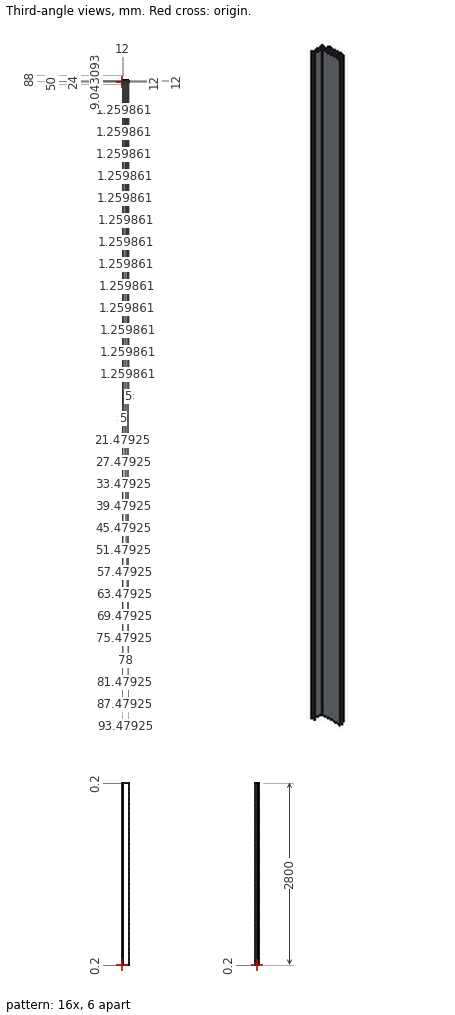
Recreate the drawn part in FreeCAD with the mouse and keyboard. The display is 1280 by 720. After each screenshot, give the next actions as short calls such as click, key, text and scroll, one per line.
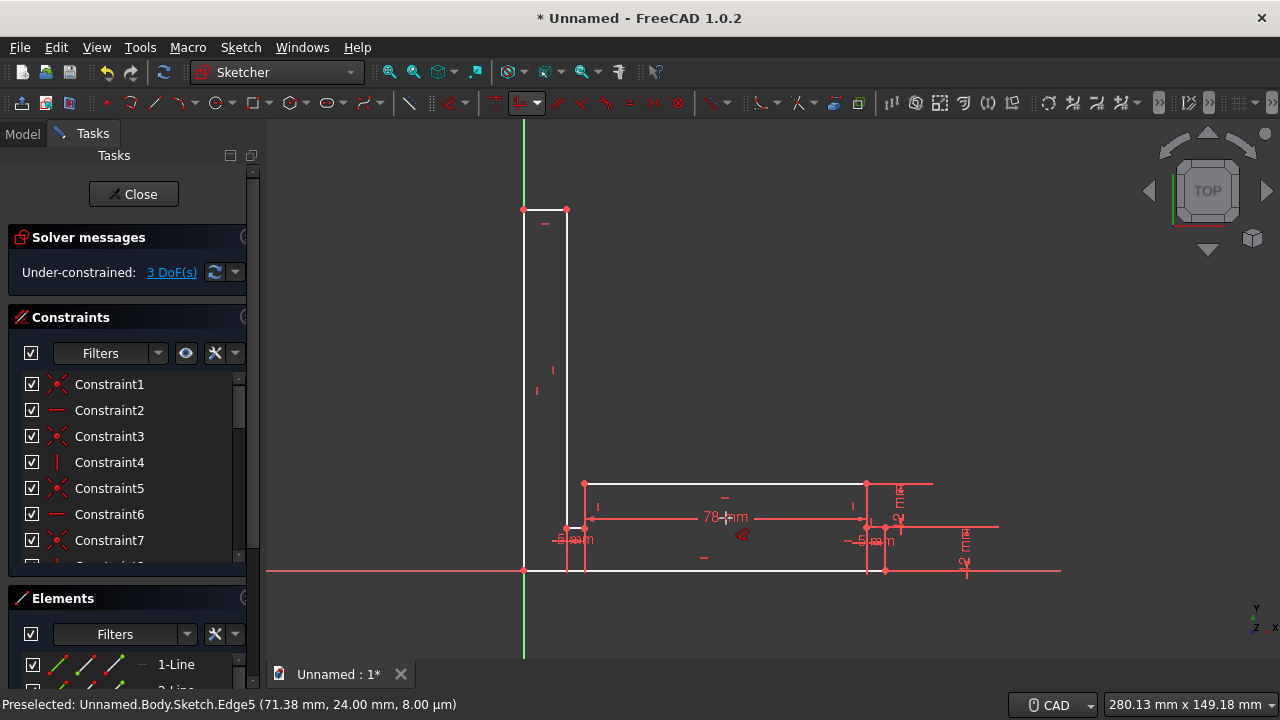
click(585, 497)
click(551, 506)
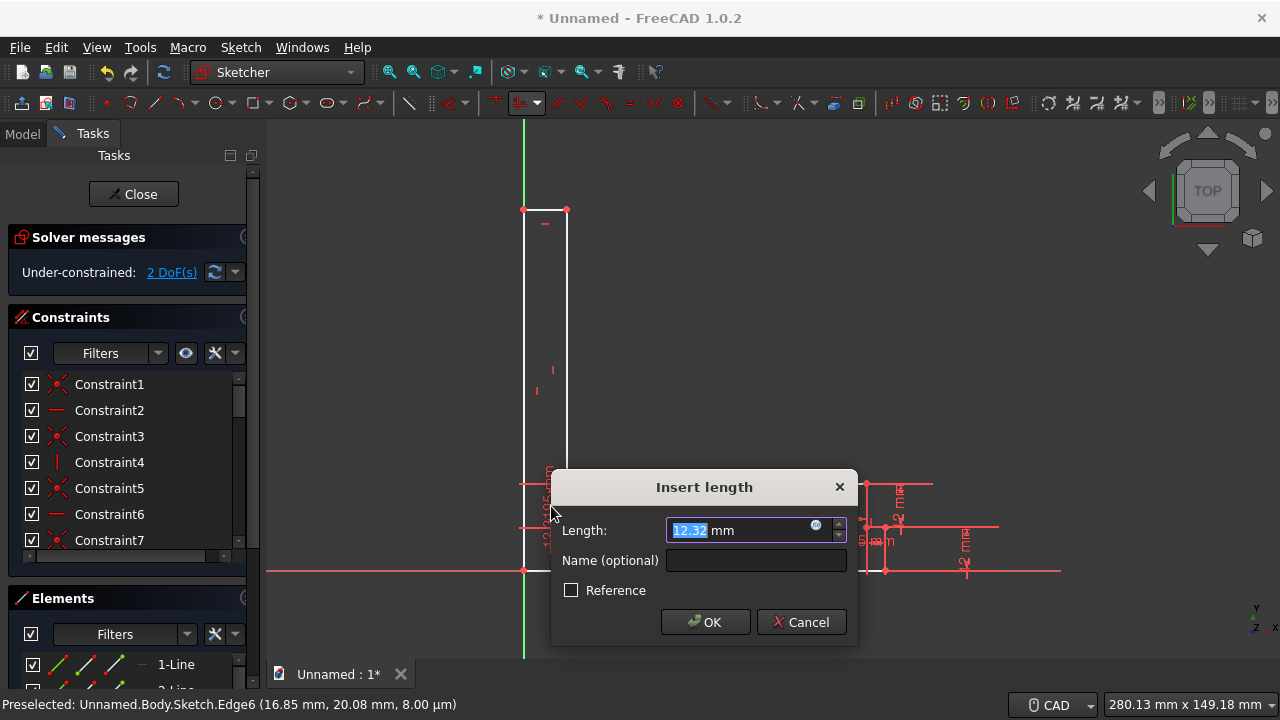
text(12)
key(Return)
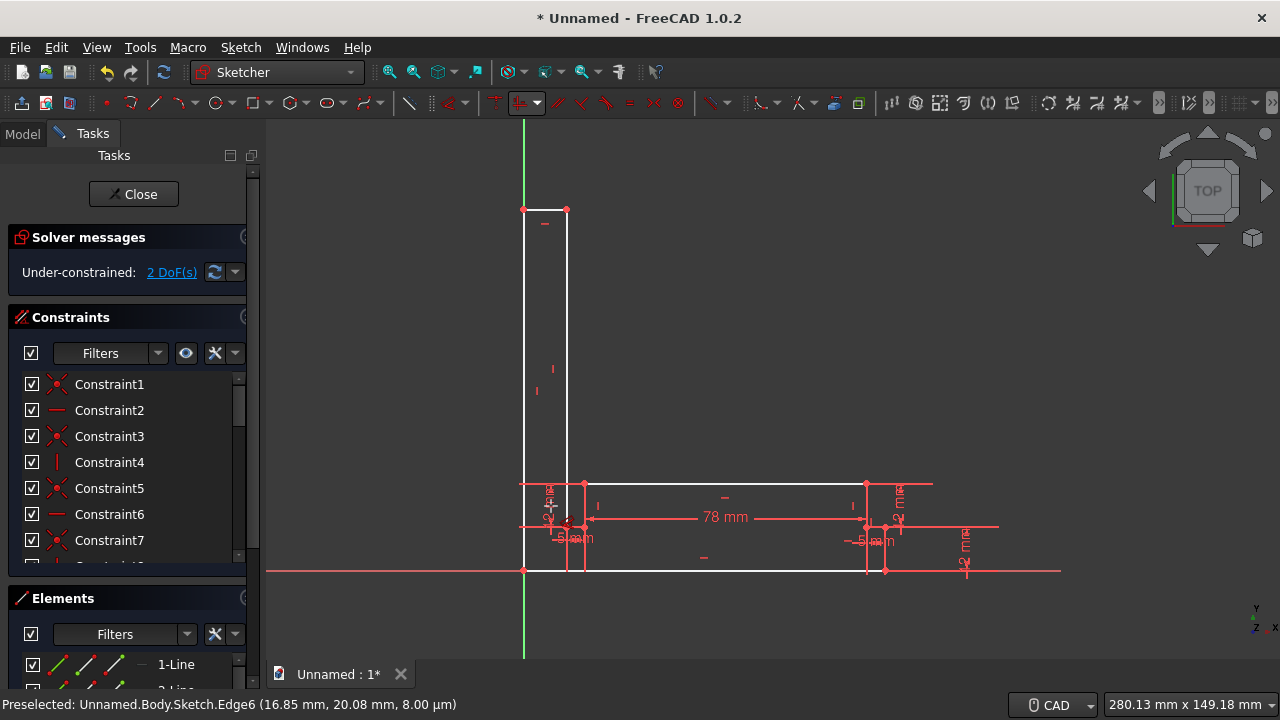
click(567, 432)
click(601, 368)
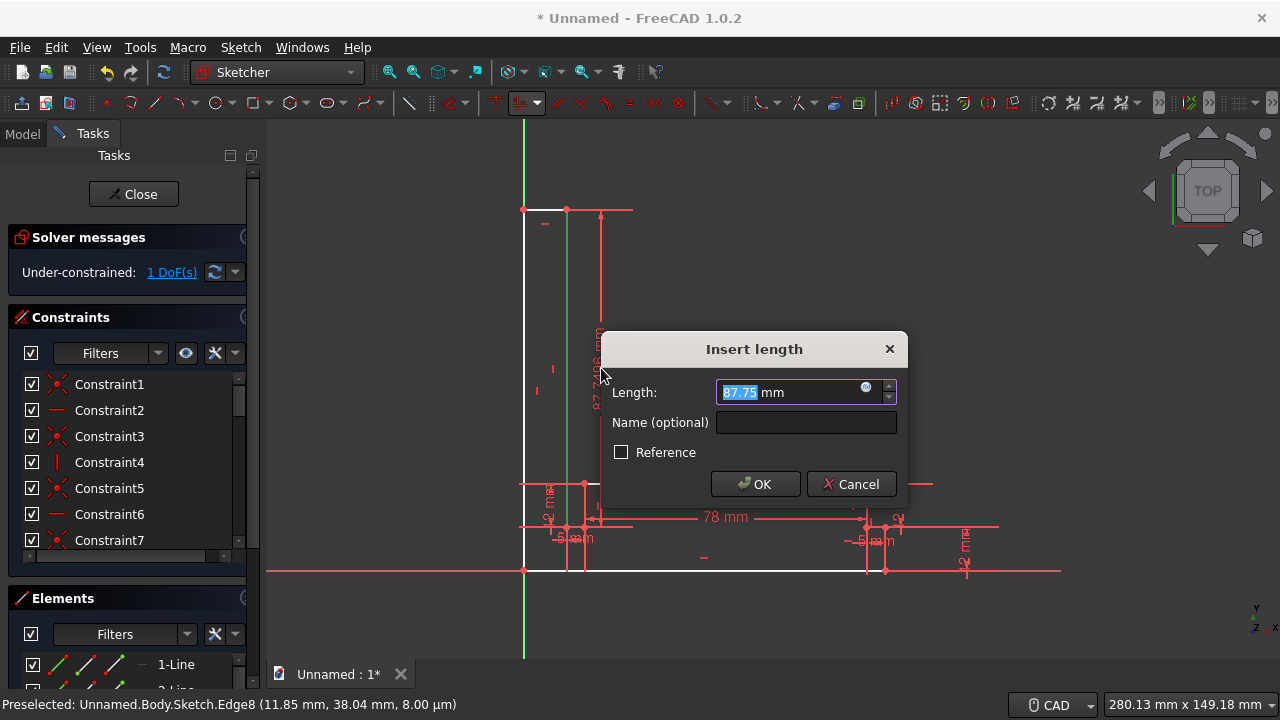
text(88)
key(Return)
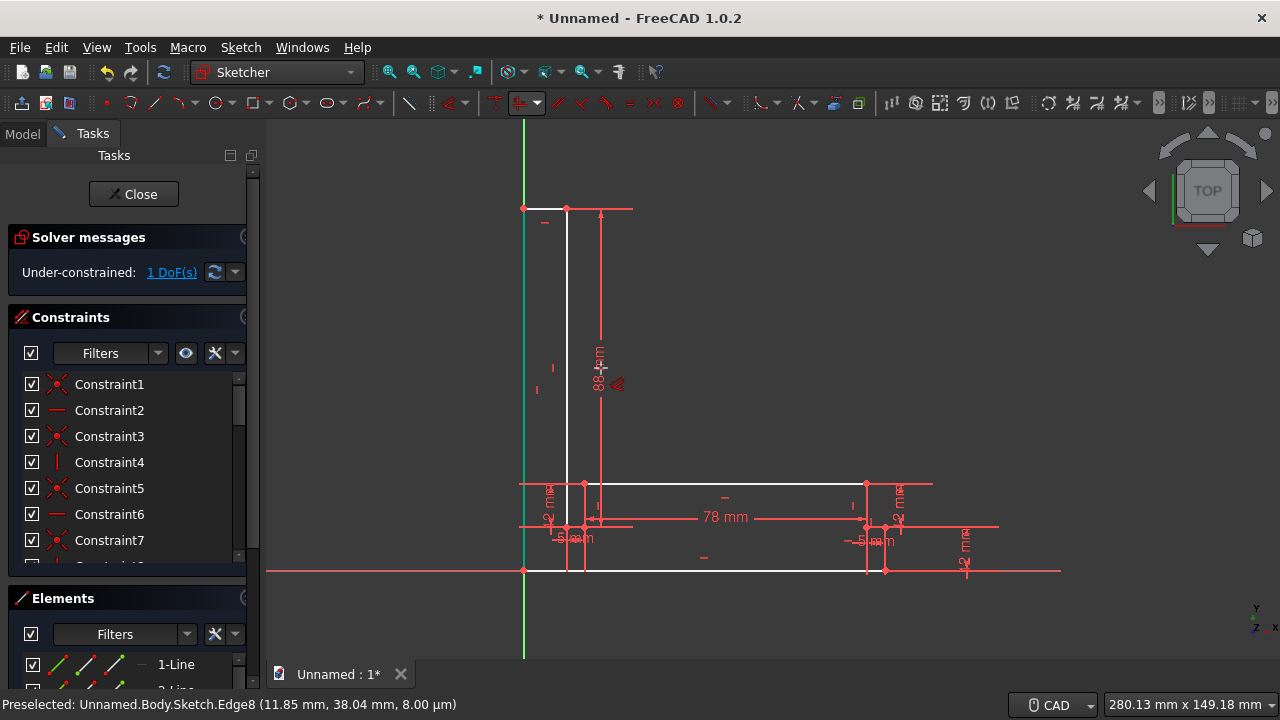
click(554, 209)
click(545, 175)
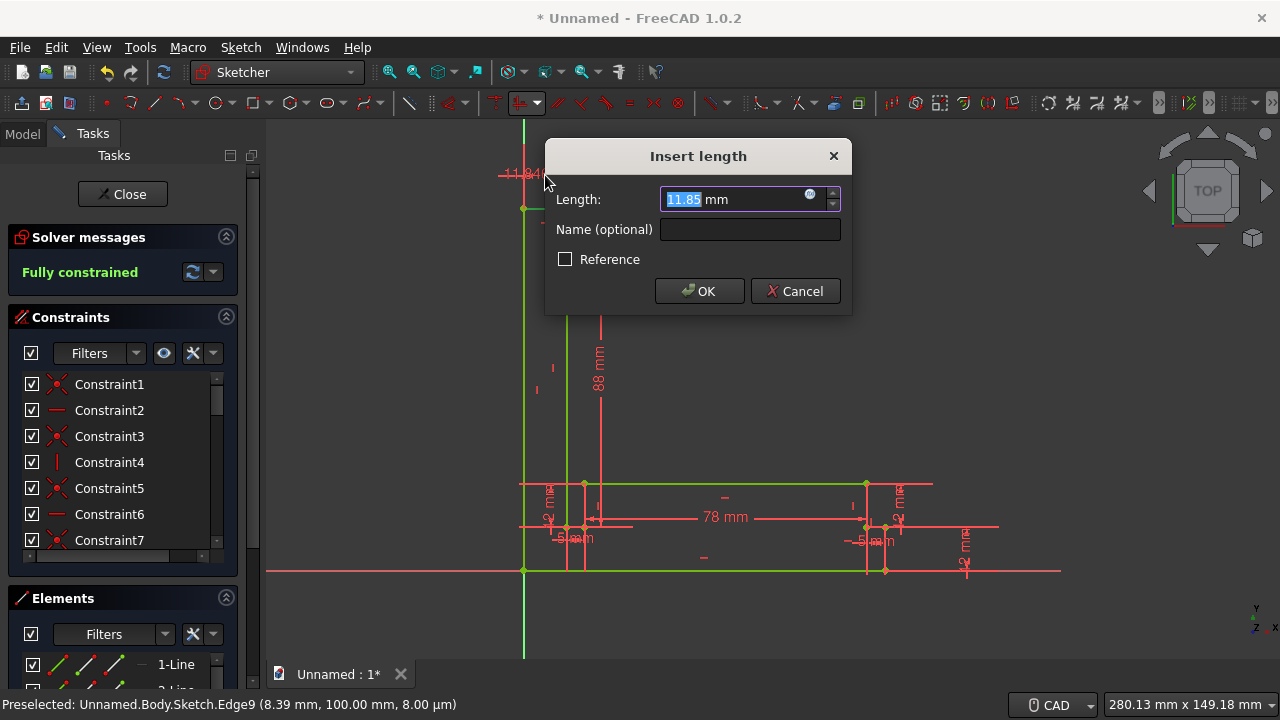
text(12)
key(Return)
key(Escape)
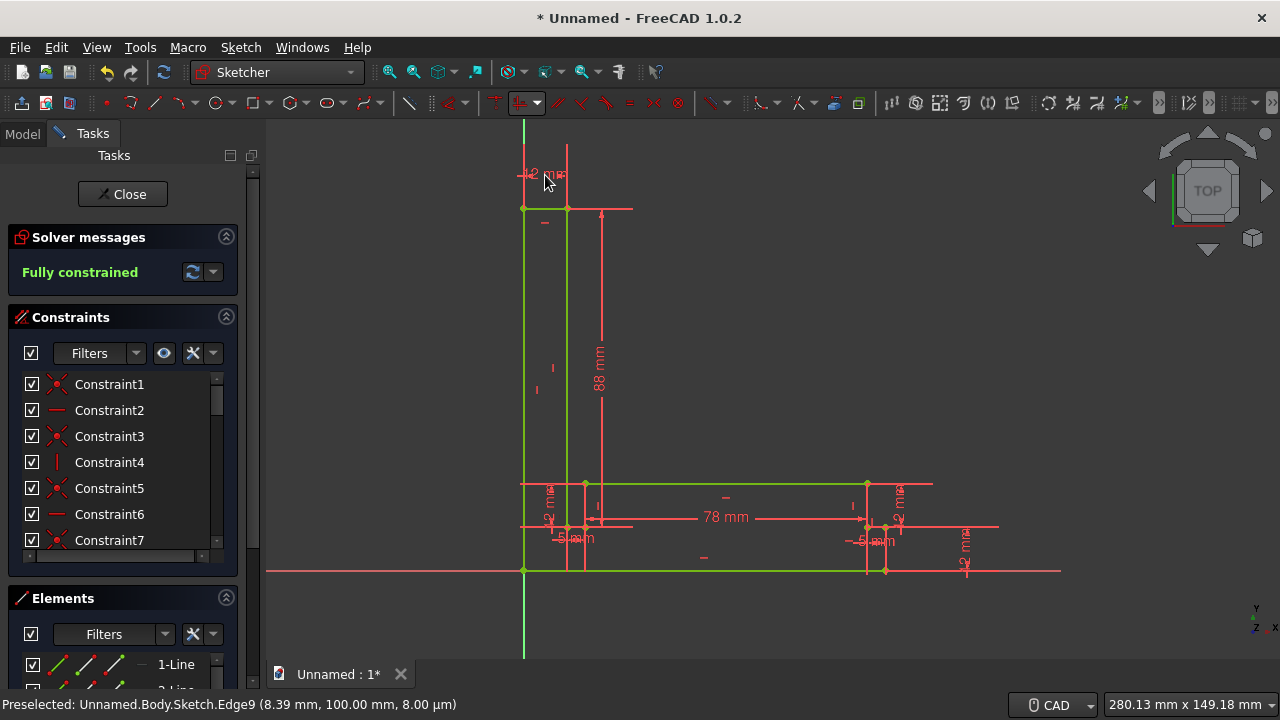
click(123, 194)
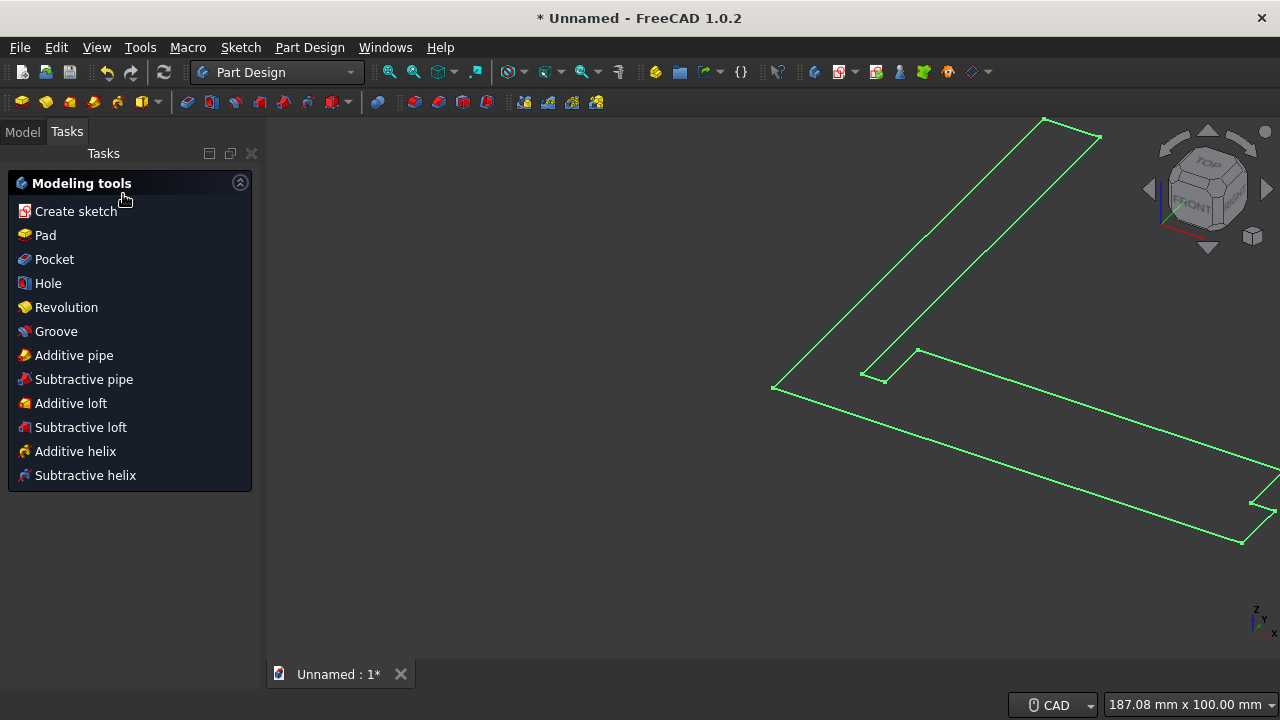
click(22, 102)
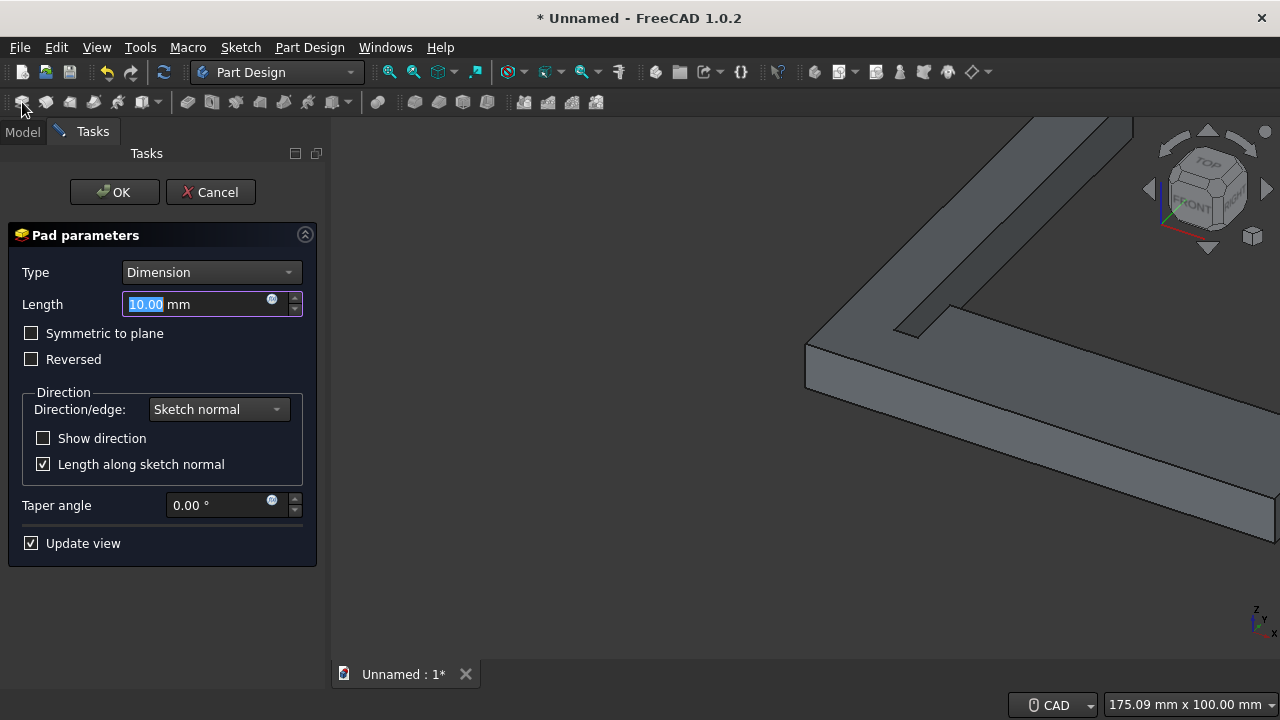
text(2800)
key(Tab)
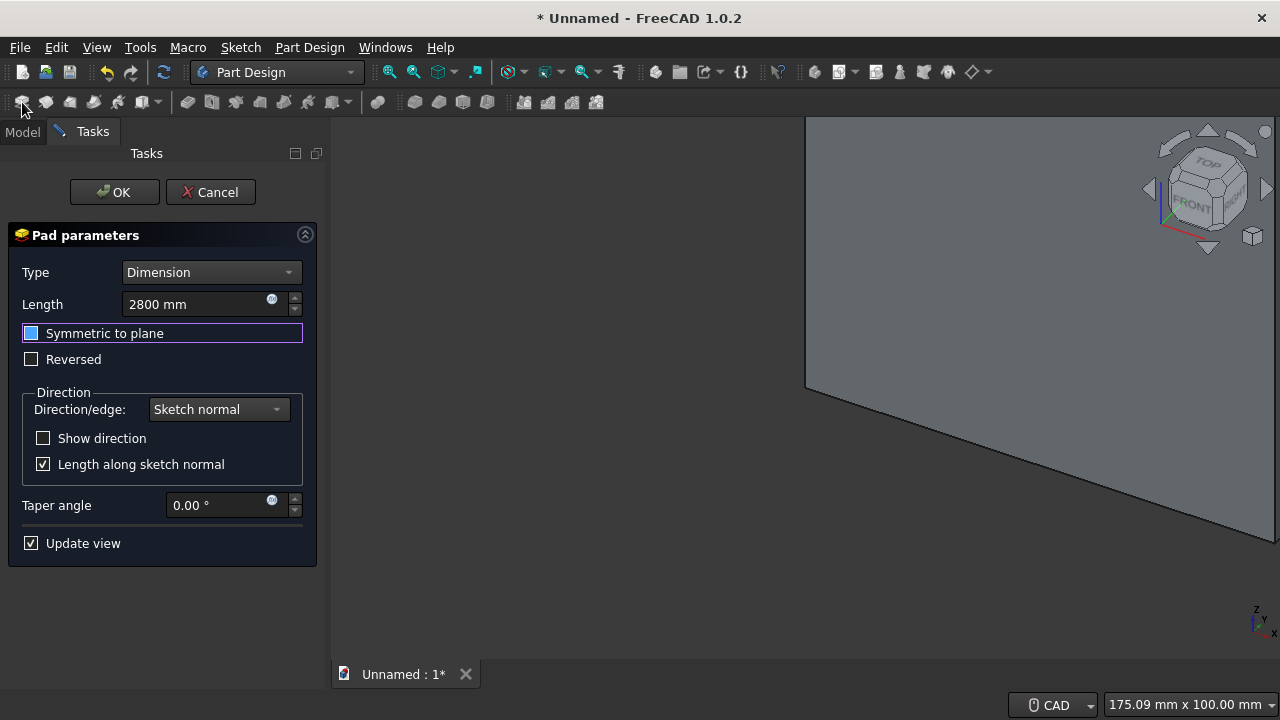
click(115, 192)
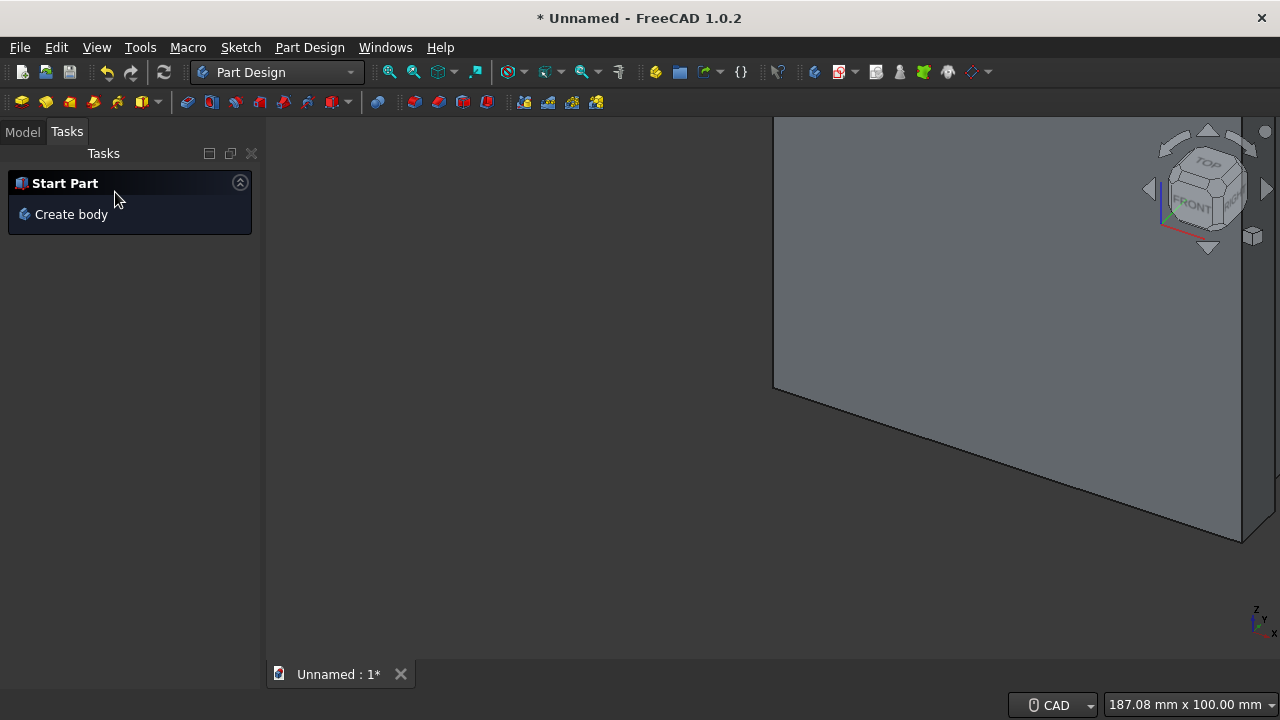
click(390, 72)